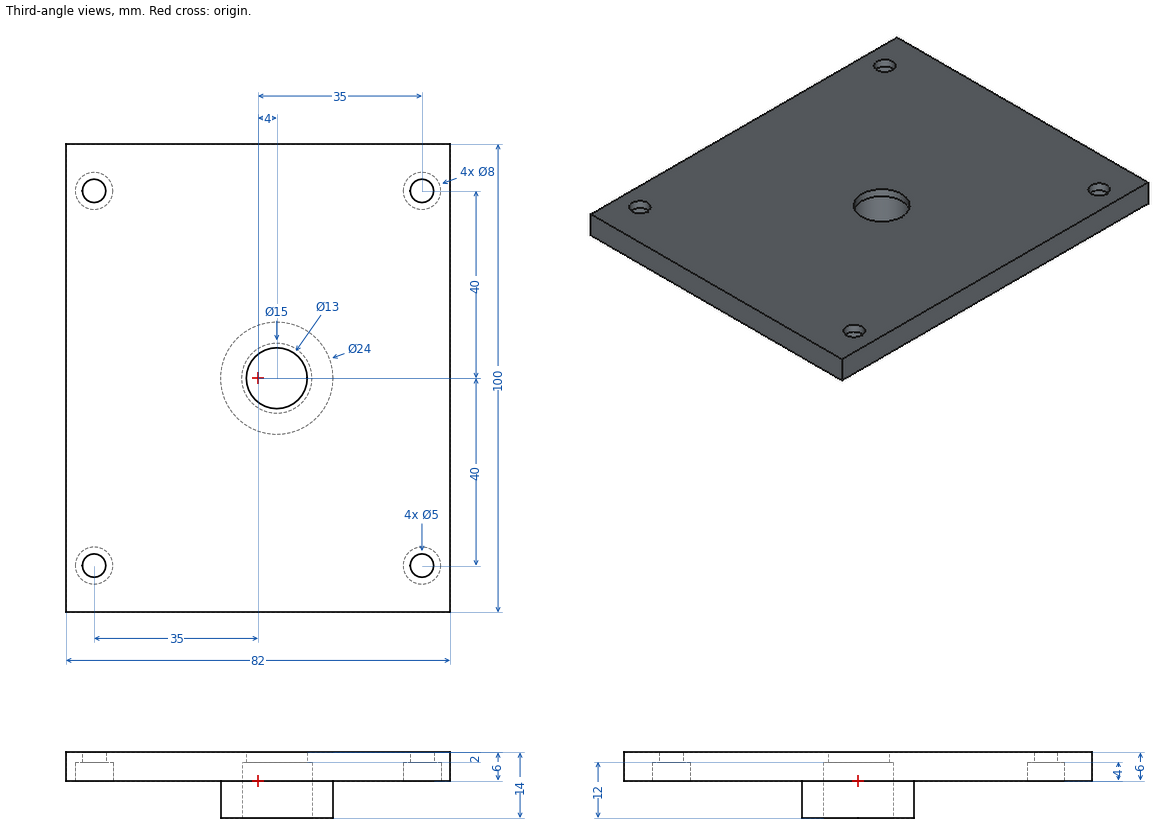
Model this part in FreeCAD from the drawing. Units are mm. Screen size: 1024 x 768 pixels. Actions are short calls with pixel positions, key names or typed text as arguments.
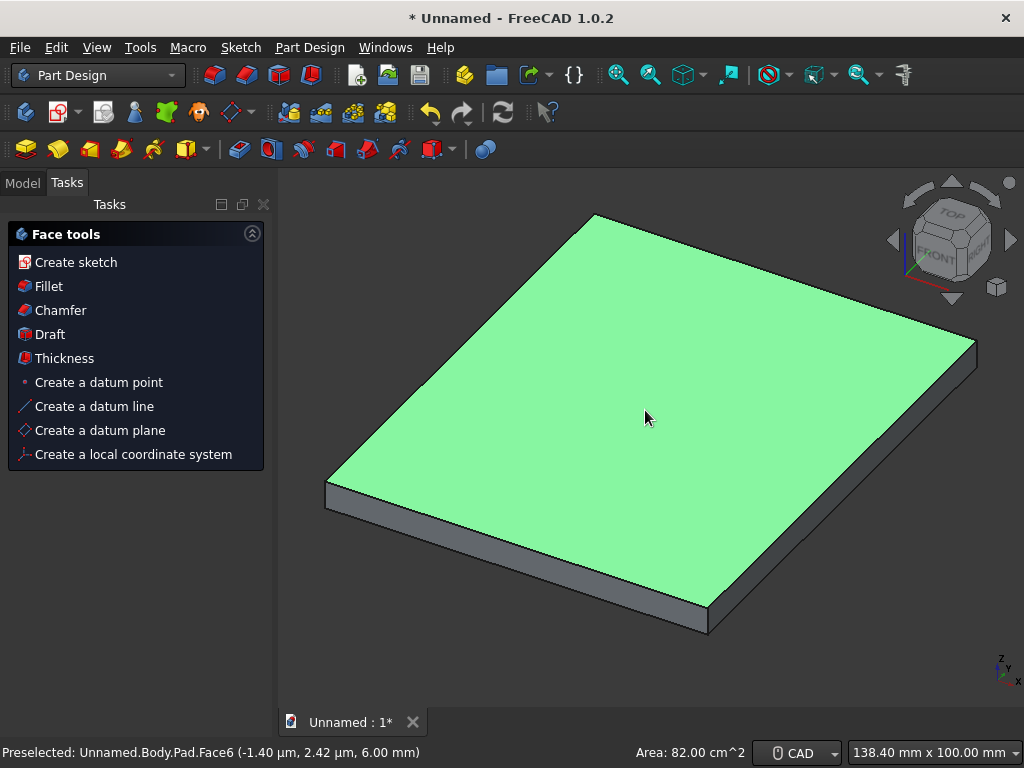
click(58, 112)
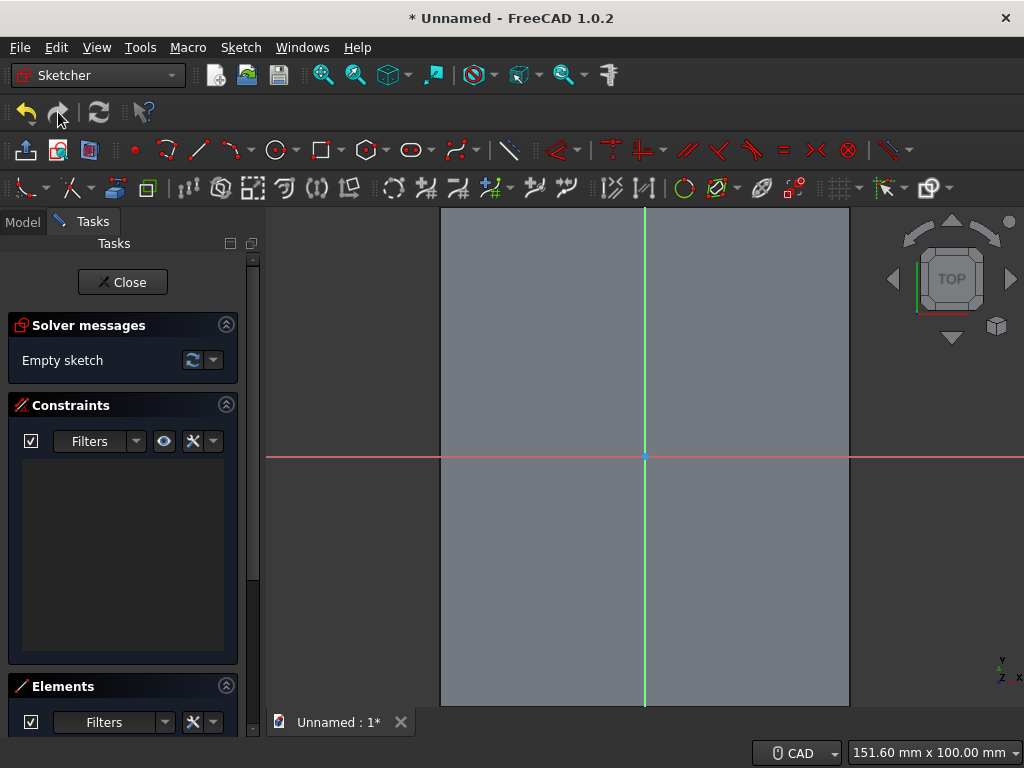
scroll(717, 457, up, 5)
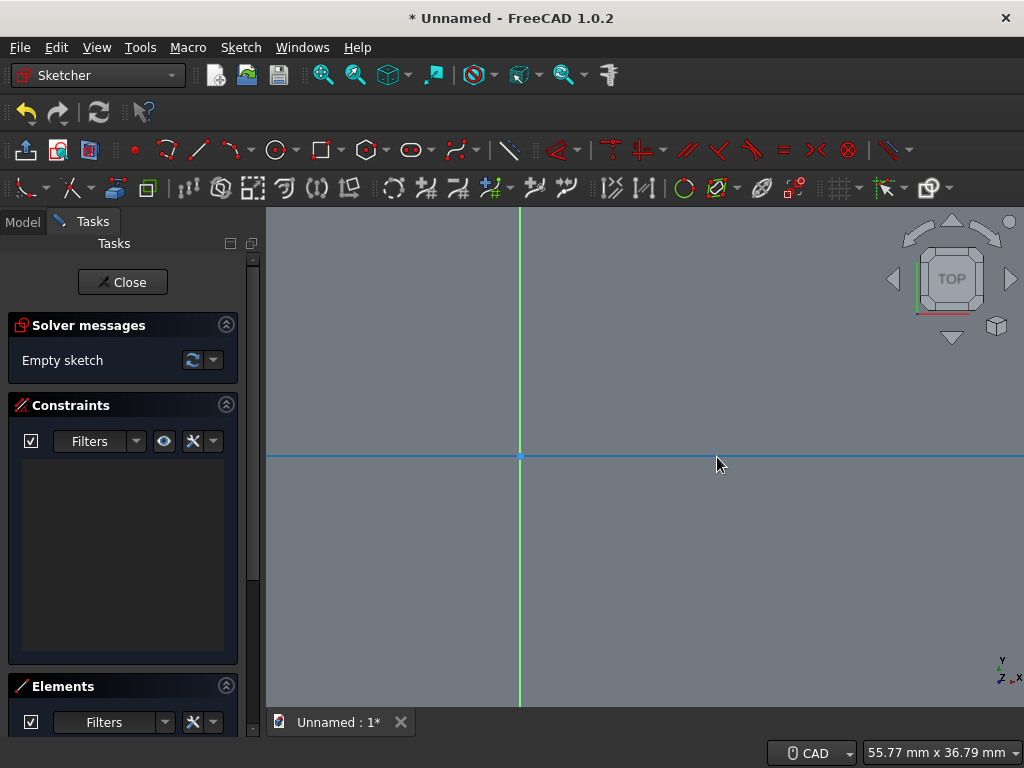
click(276, 150)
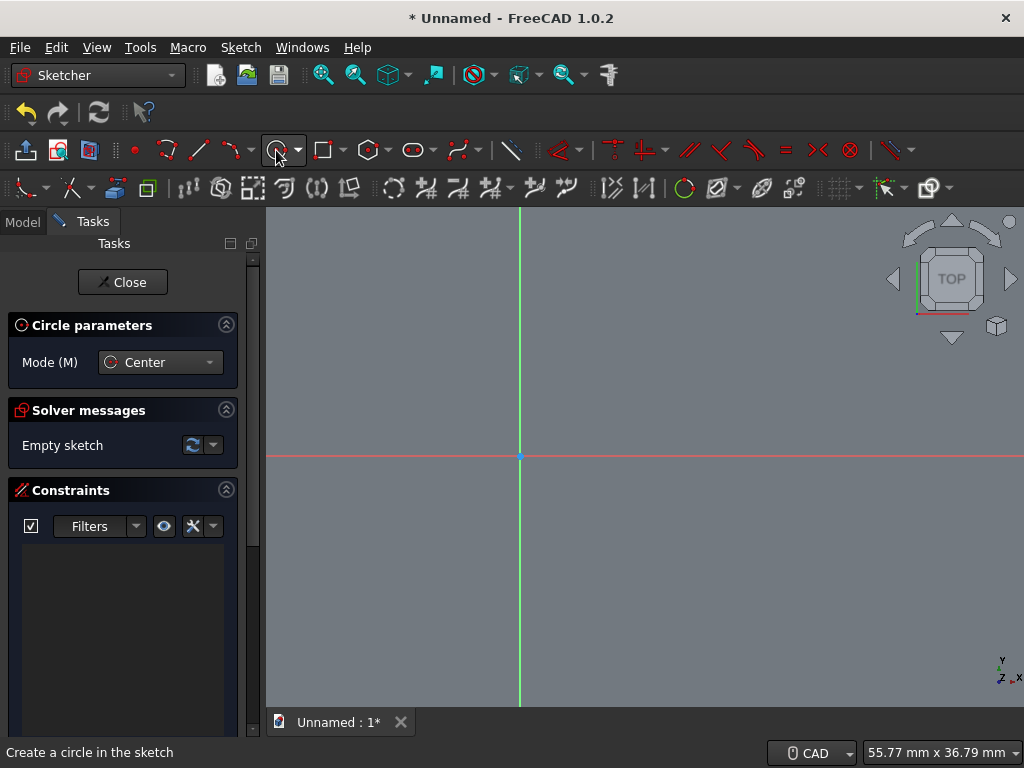
click(575, 456)
move(690, 341)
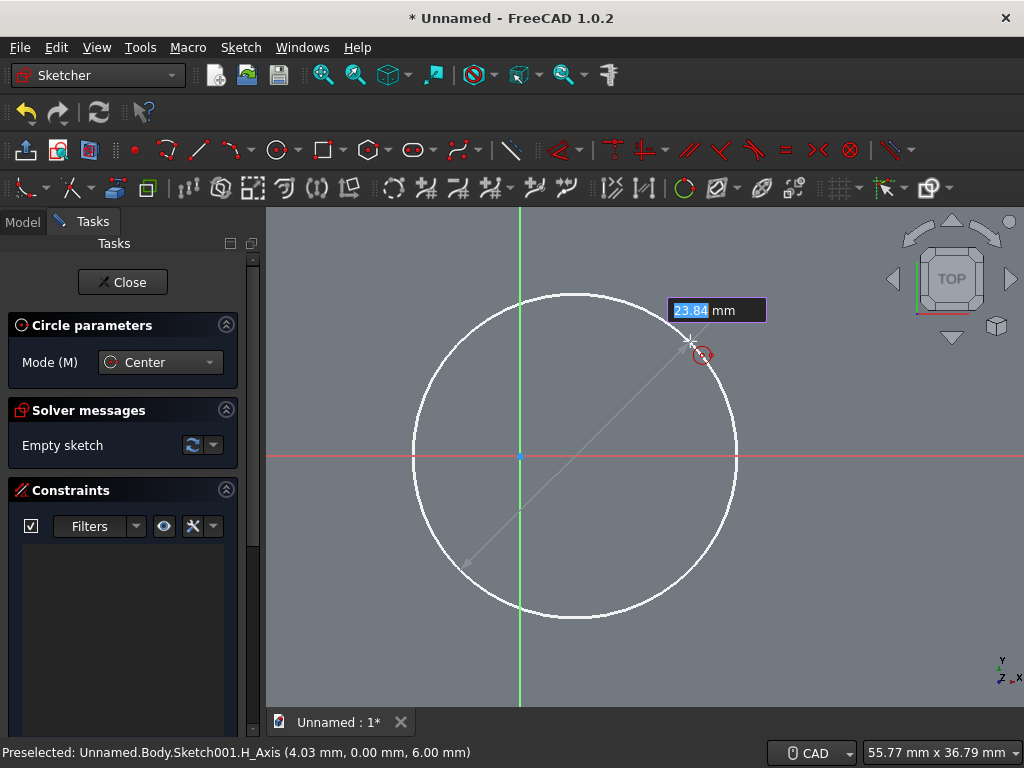
text(24)
key(Return)
key(Escape)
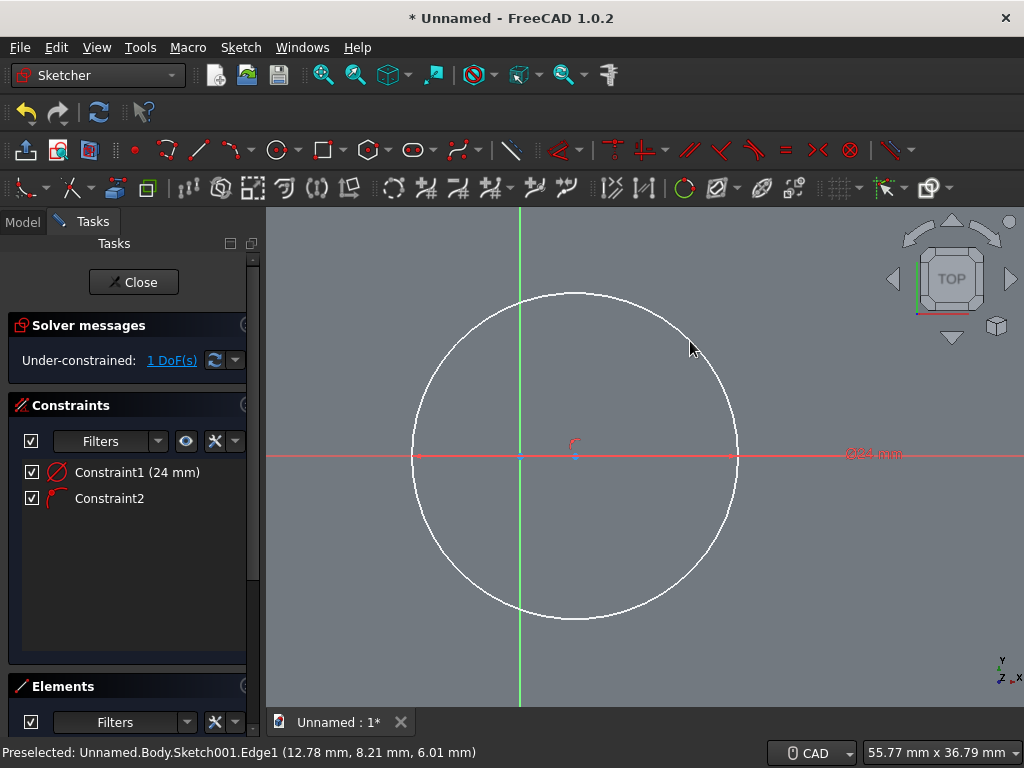
click(575, 456)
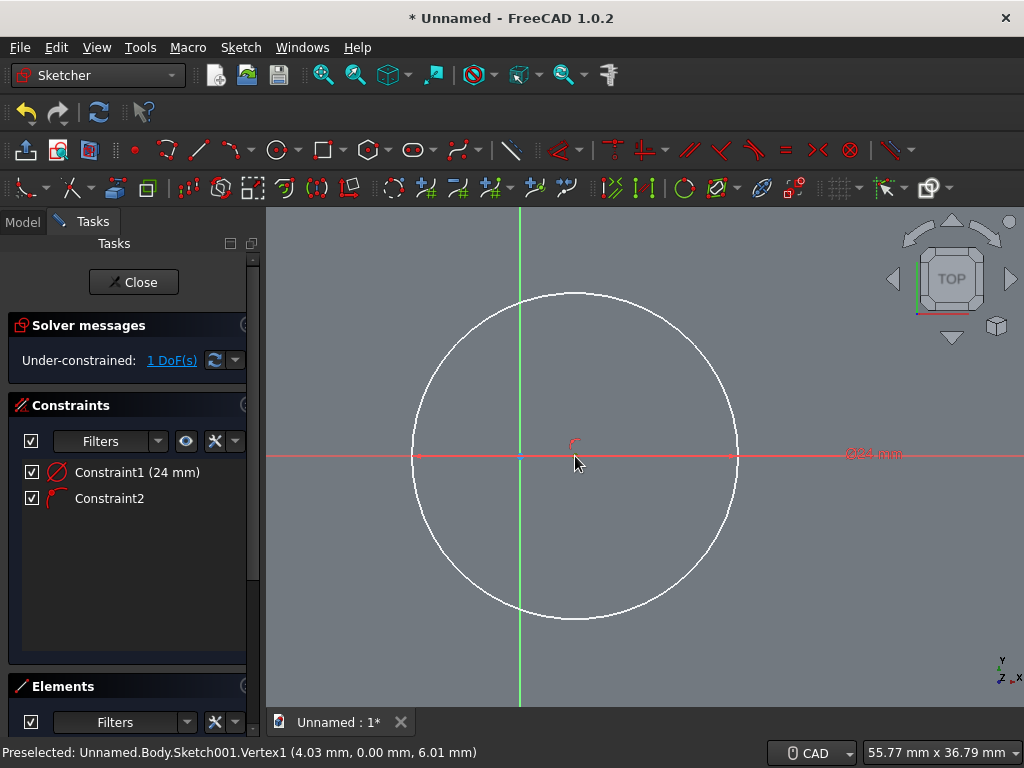
key(l)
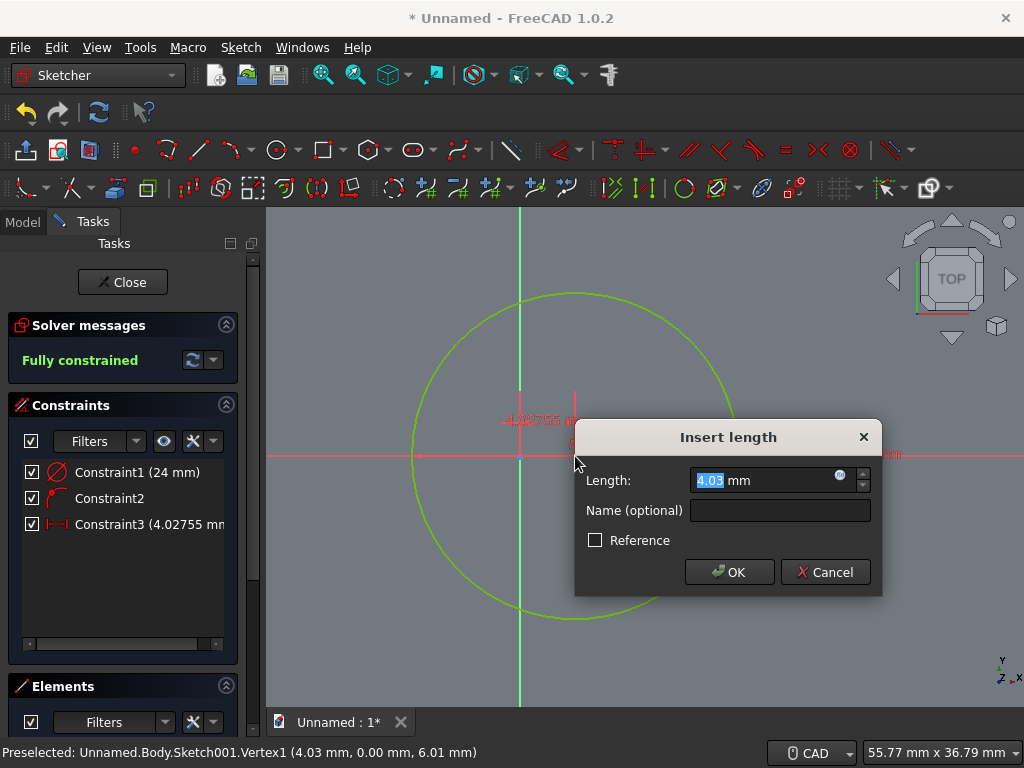
text(4)
key(Return)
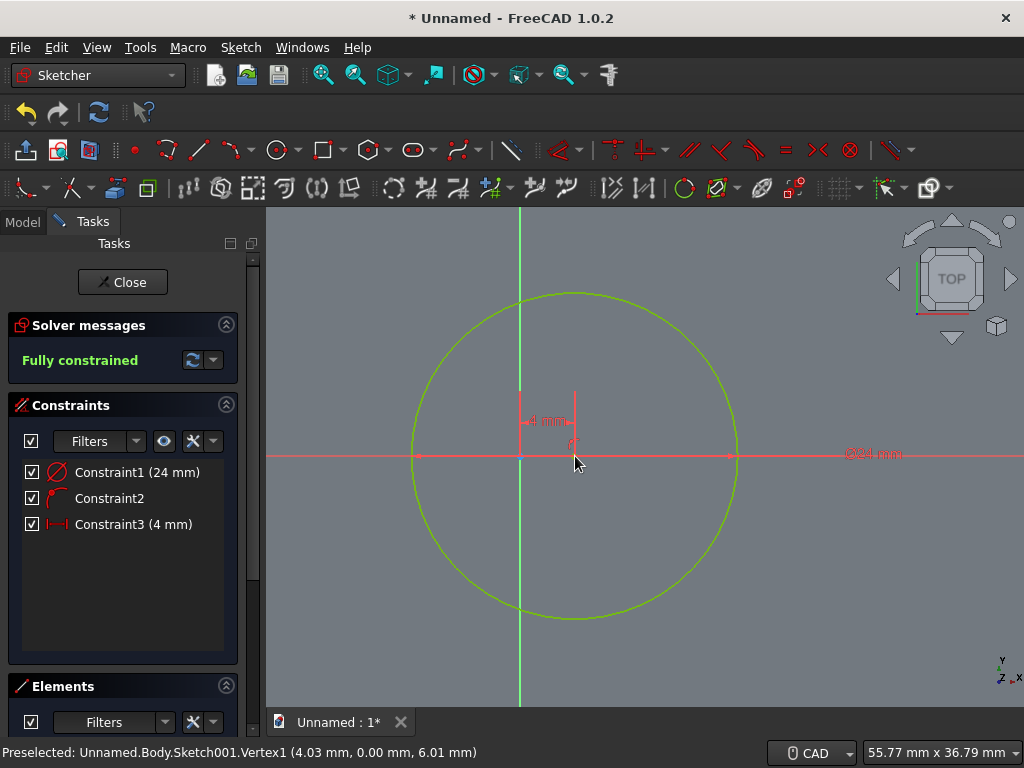
click(123, 282)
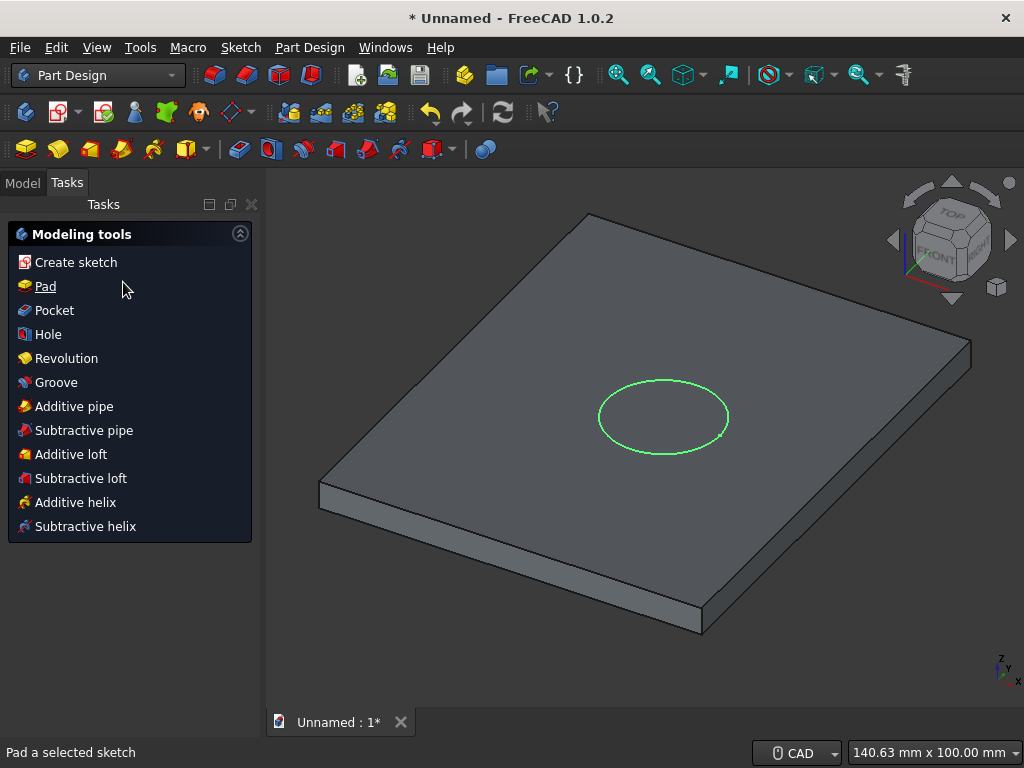
click(26, 150)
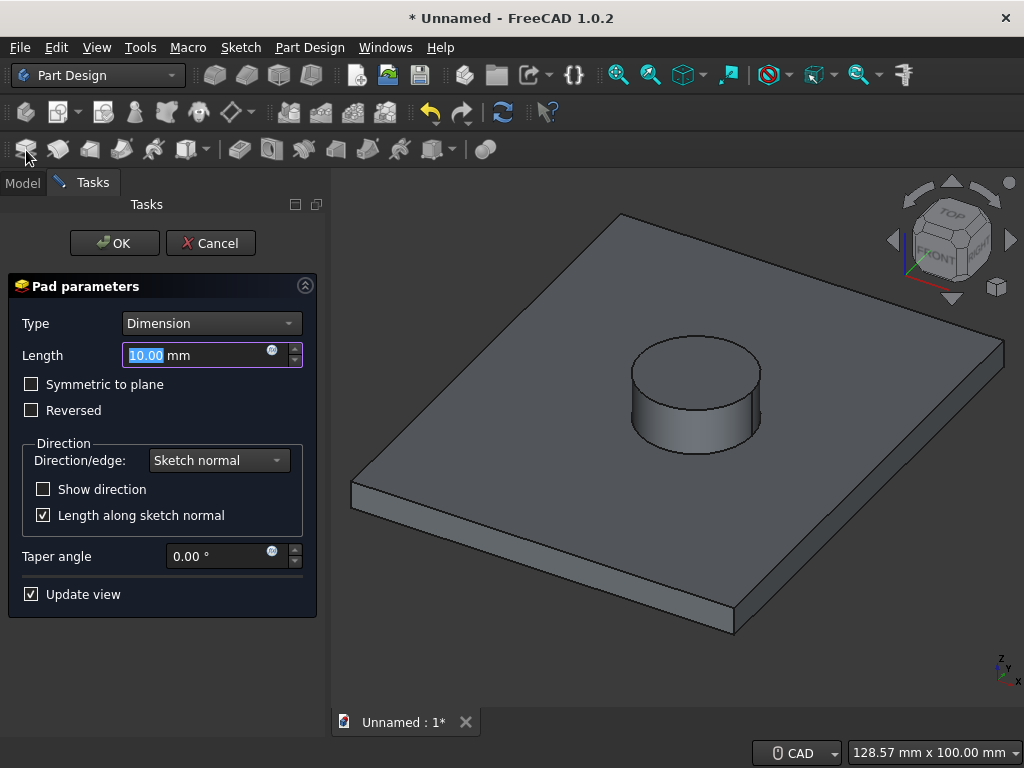
text(14)
key(Tab)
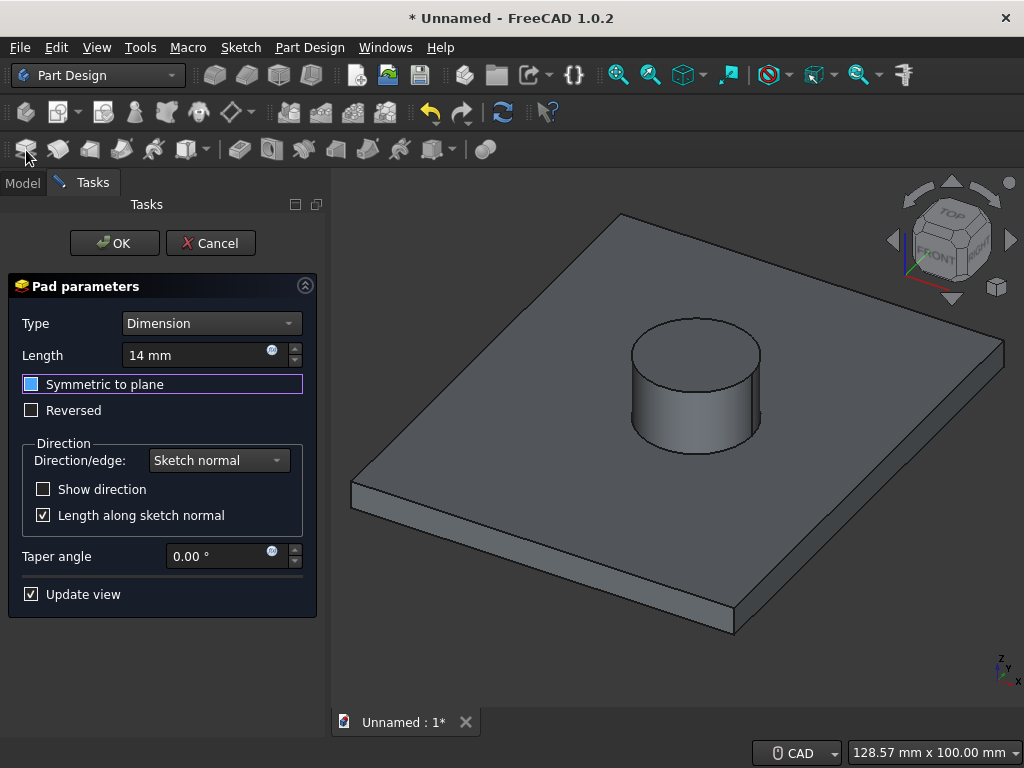
click(30, 410)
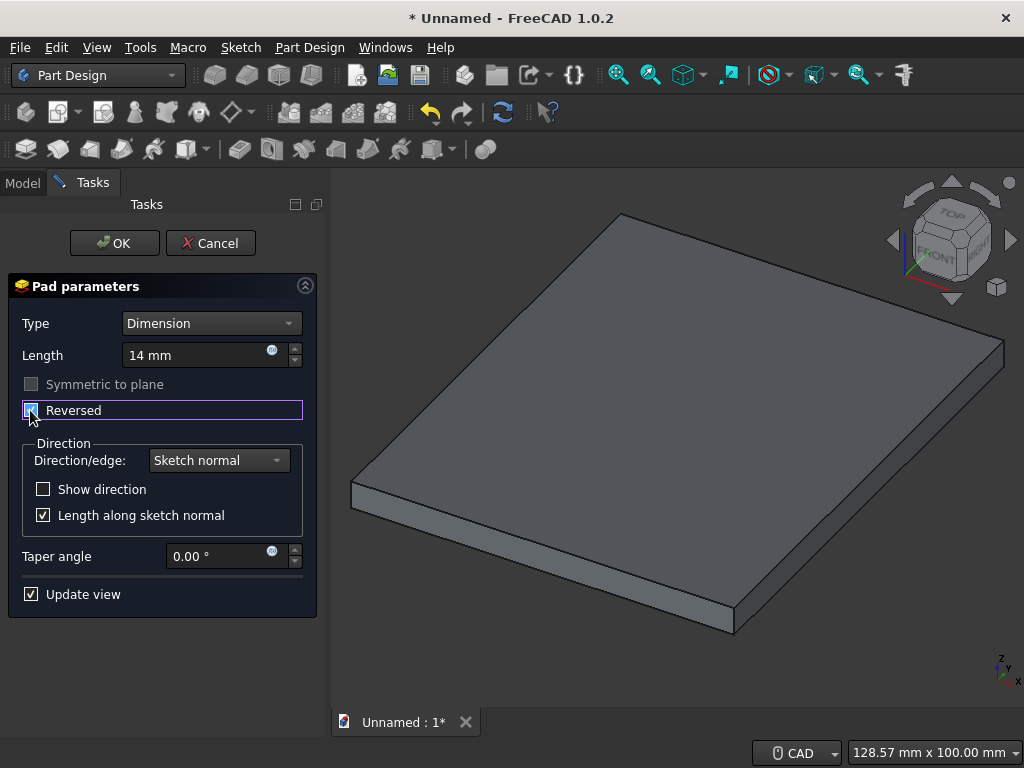
click(115, 243)